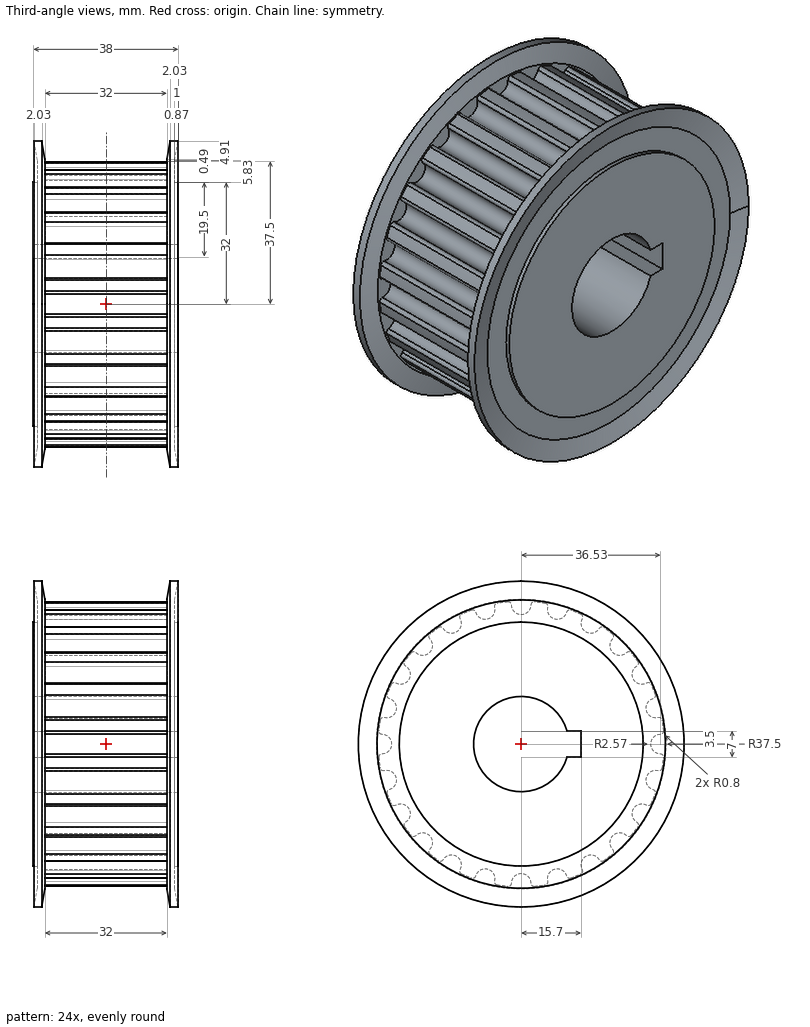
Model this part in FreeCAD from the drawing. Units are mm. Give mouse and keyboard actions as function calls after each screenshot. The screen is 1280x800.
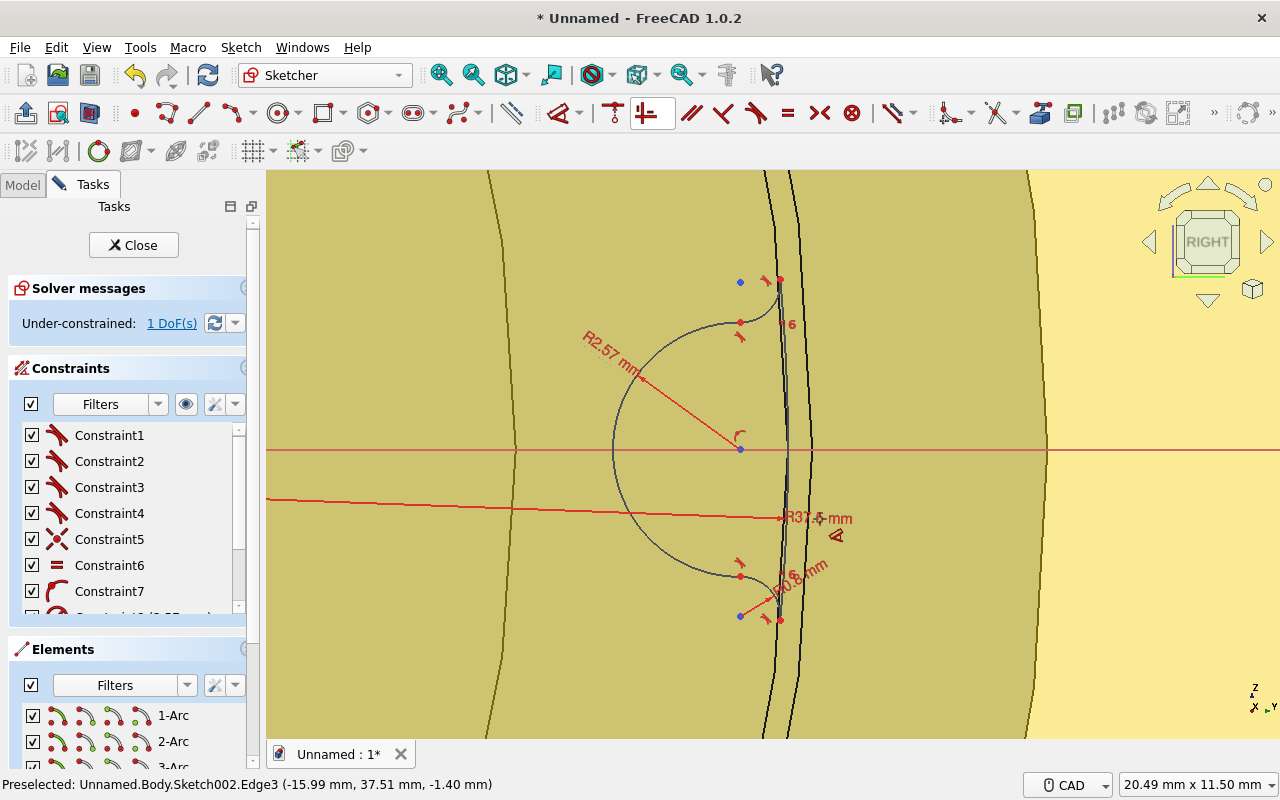
click(740, 450)
click(517, 484)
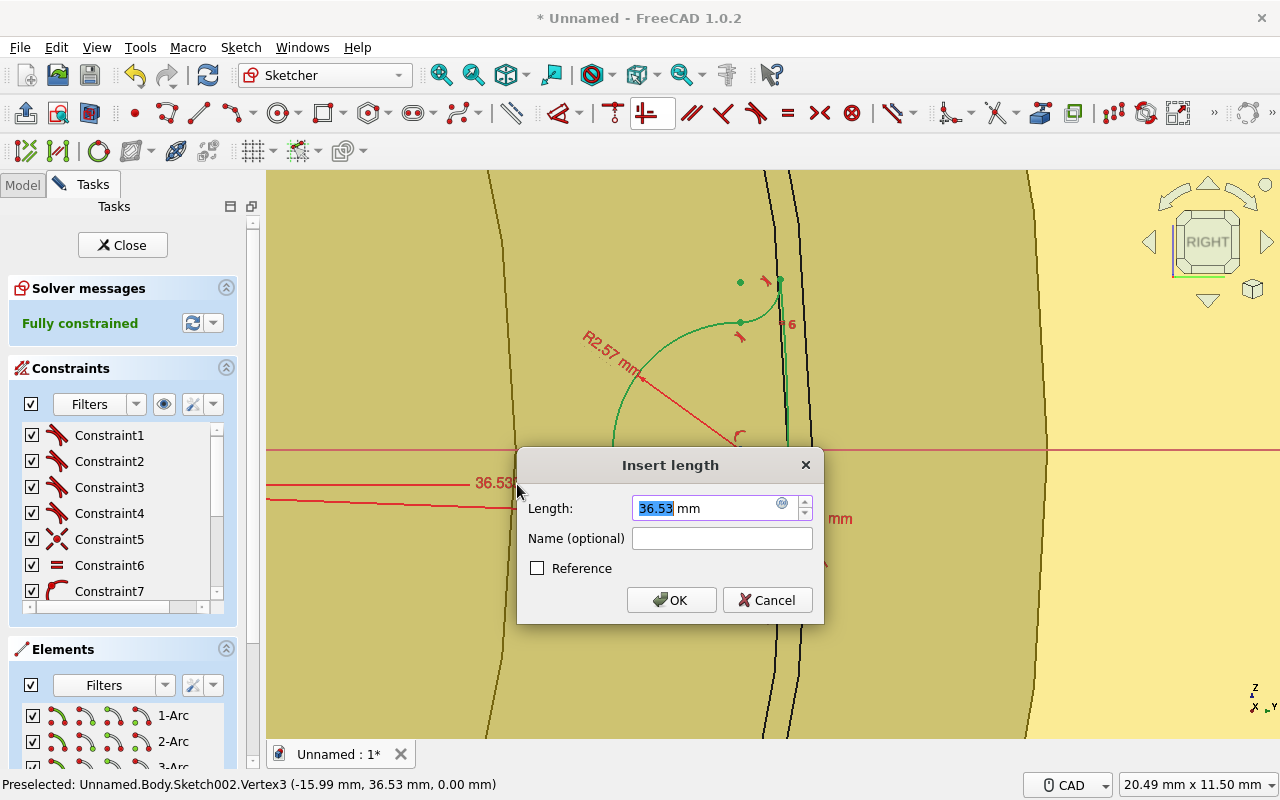
text(36.53)
key(Return)
key(Escape)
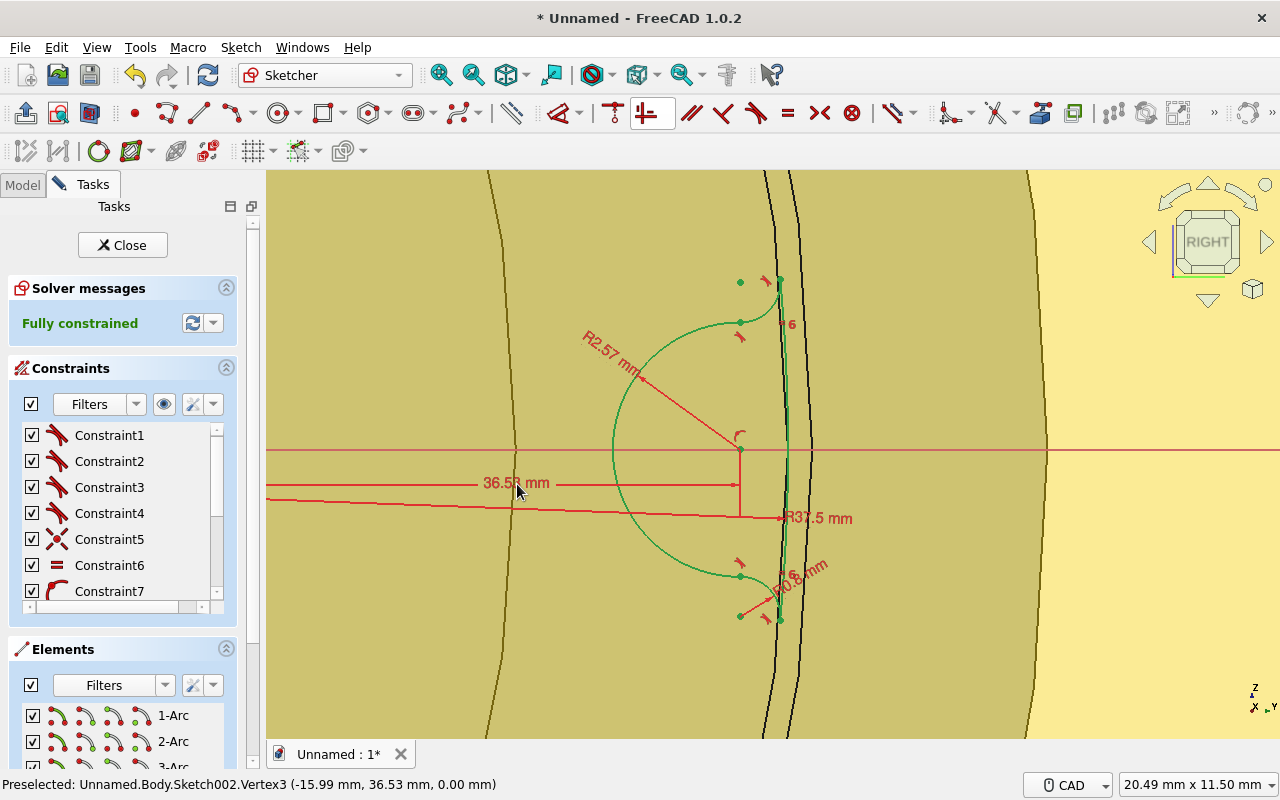
click(123, 245)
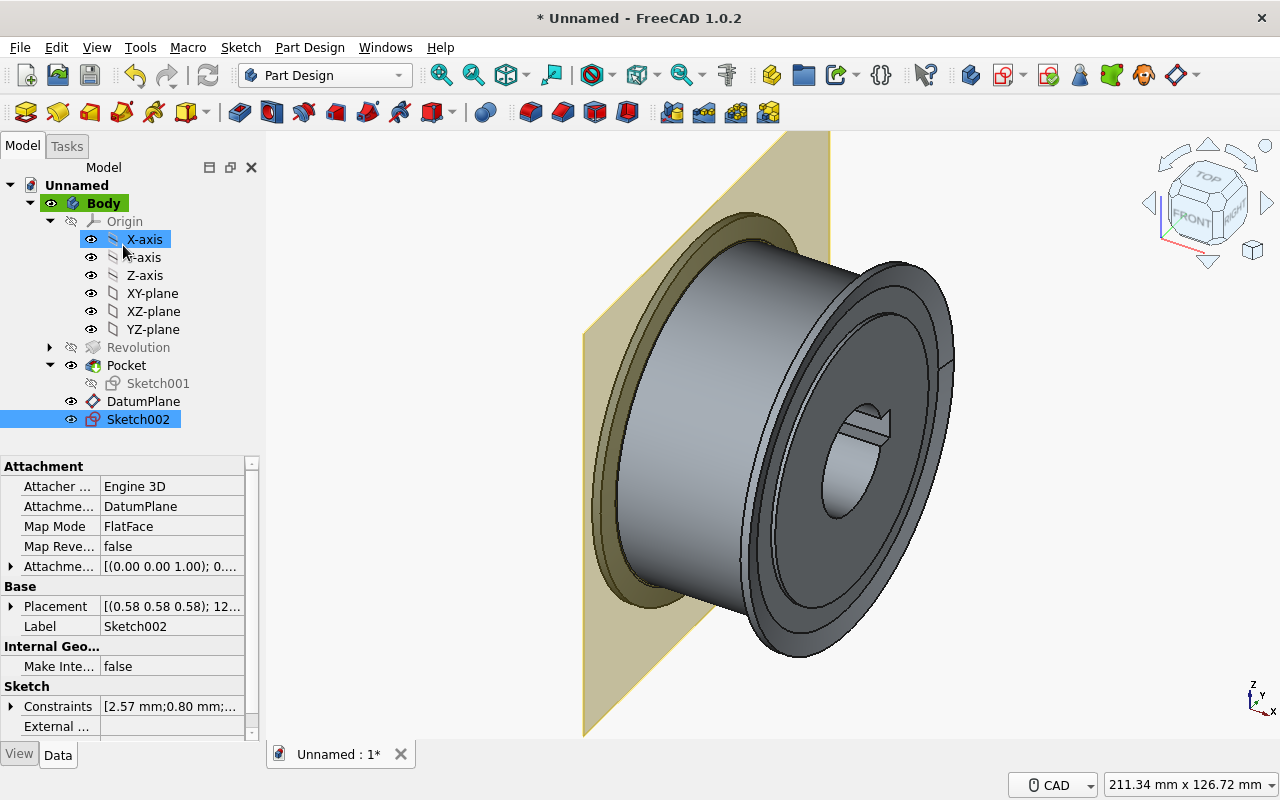
click(240, 112)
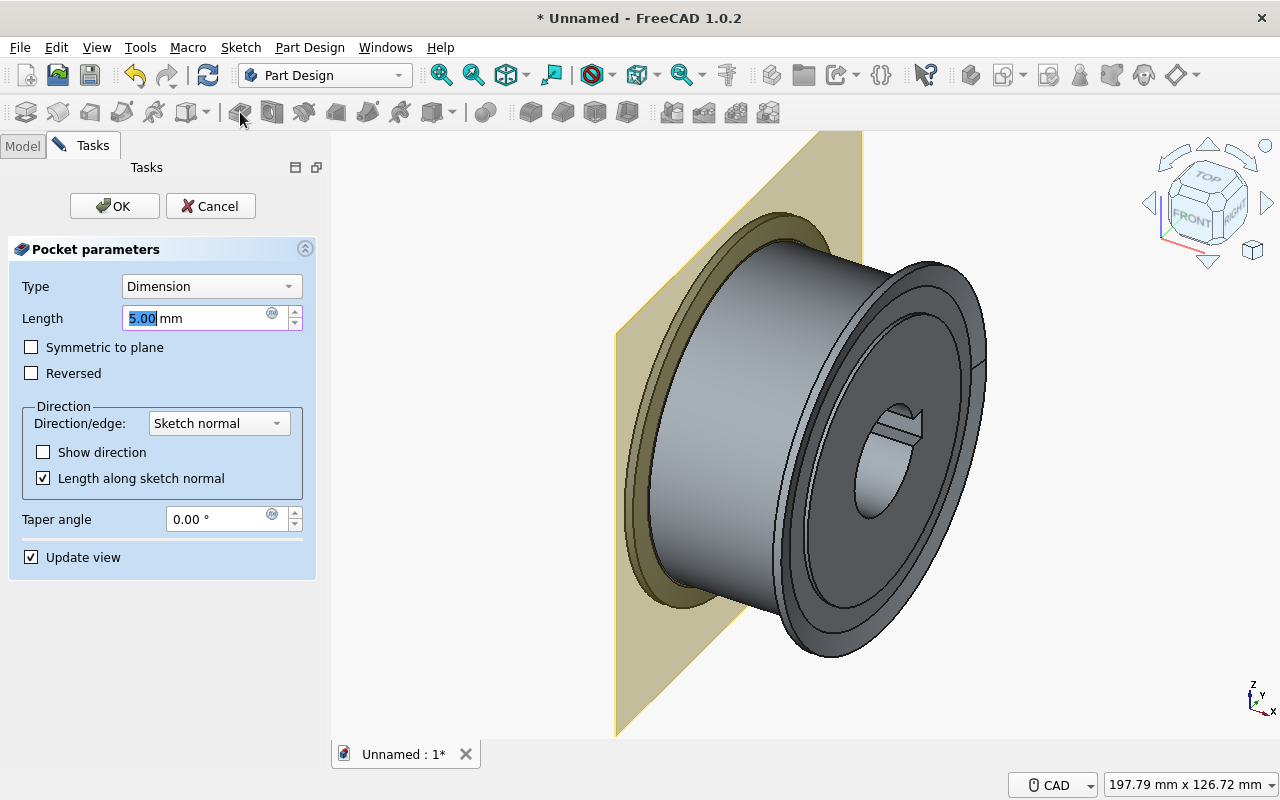
text(32)
key(Tab)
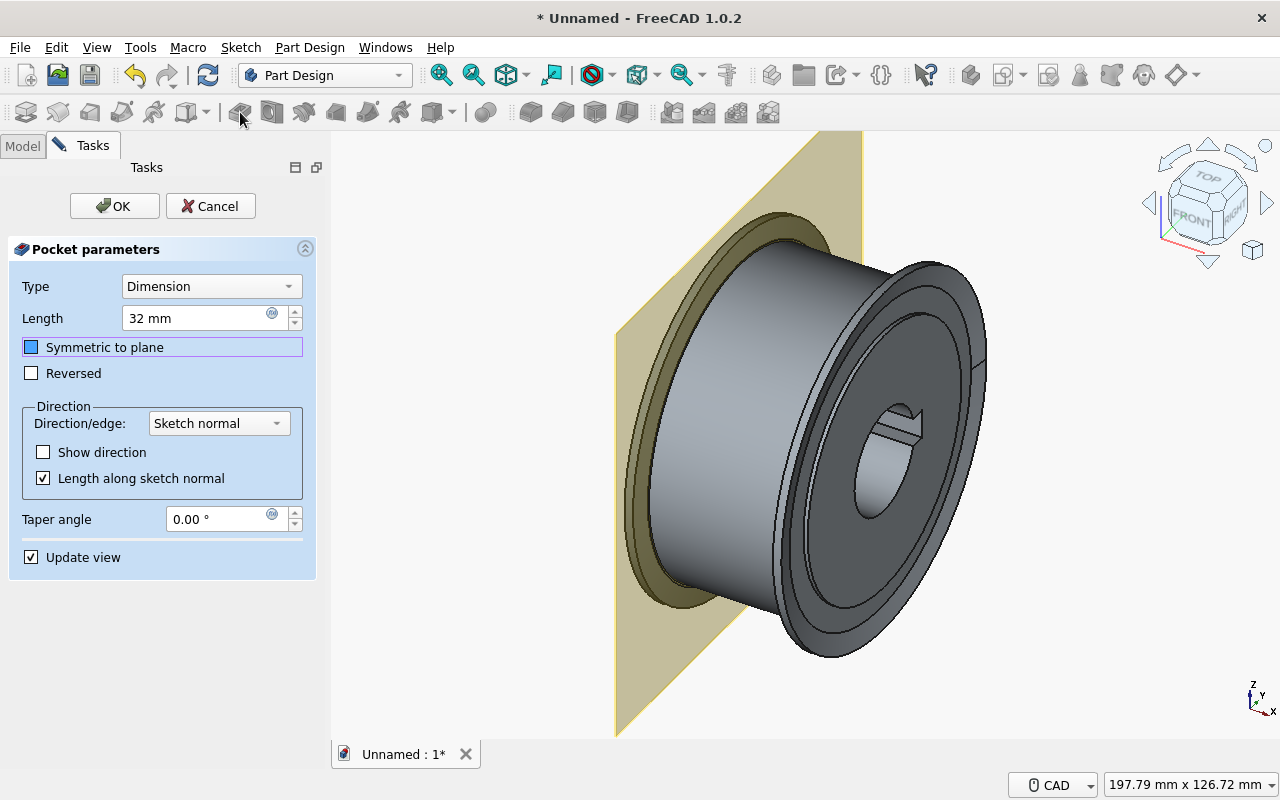
click(30, 373)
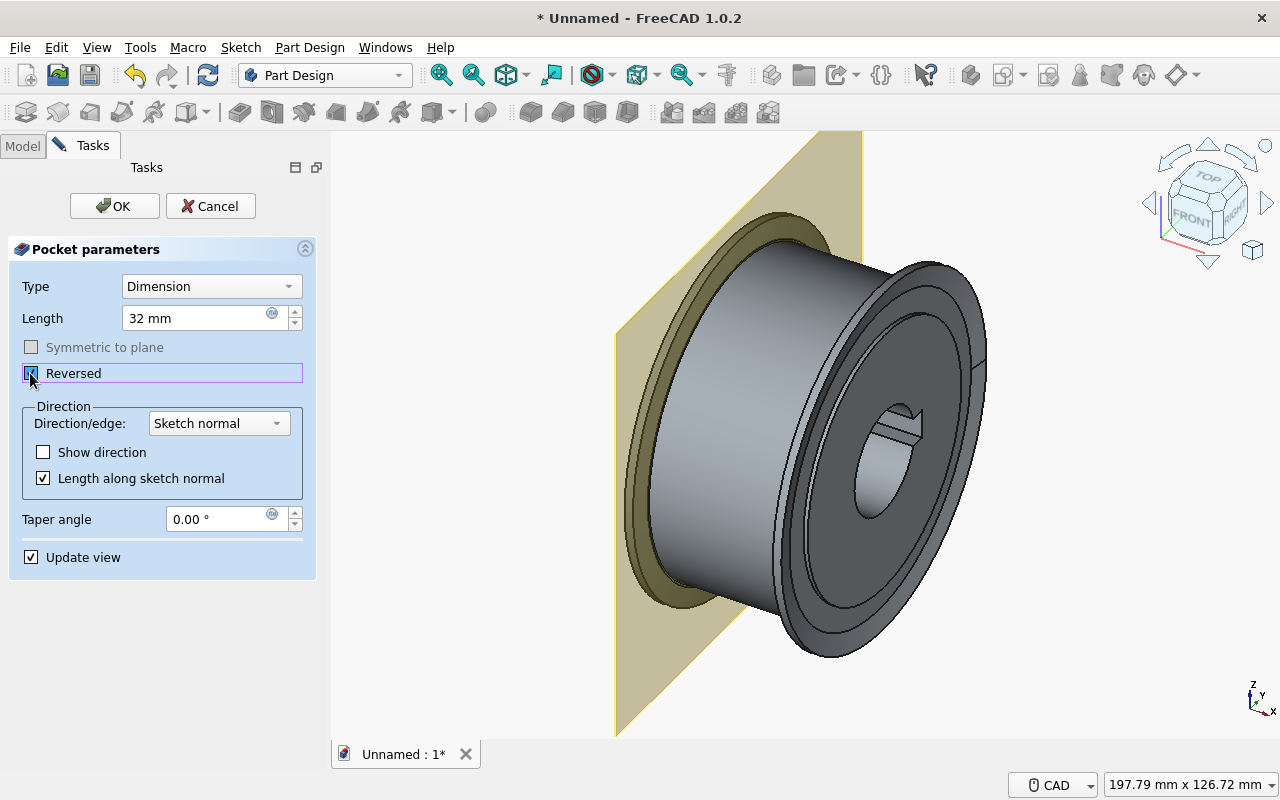
click(115, 206)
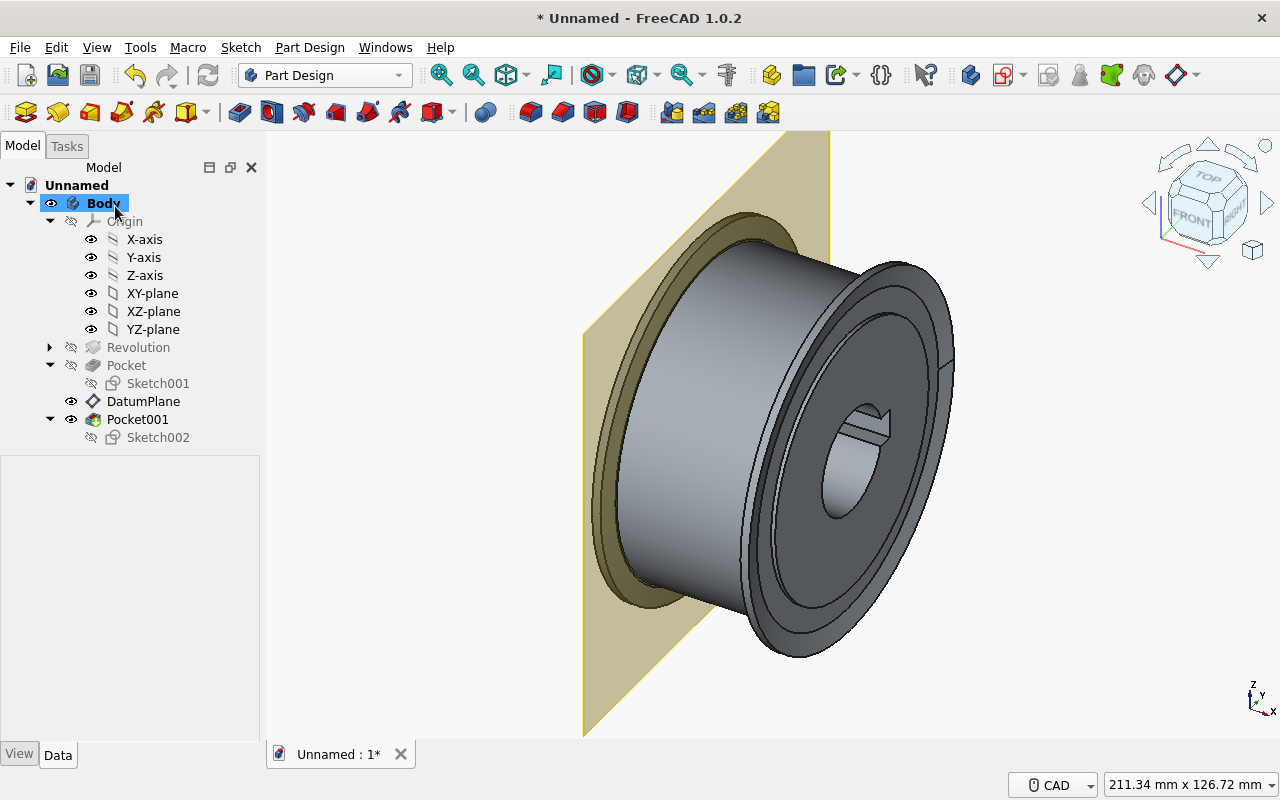
click(116, 401)
key(space)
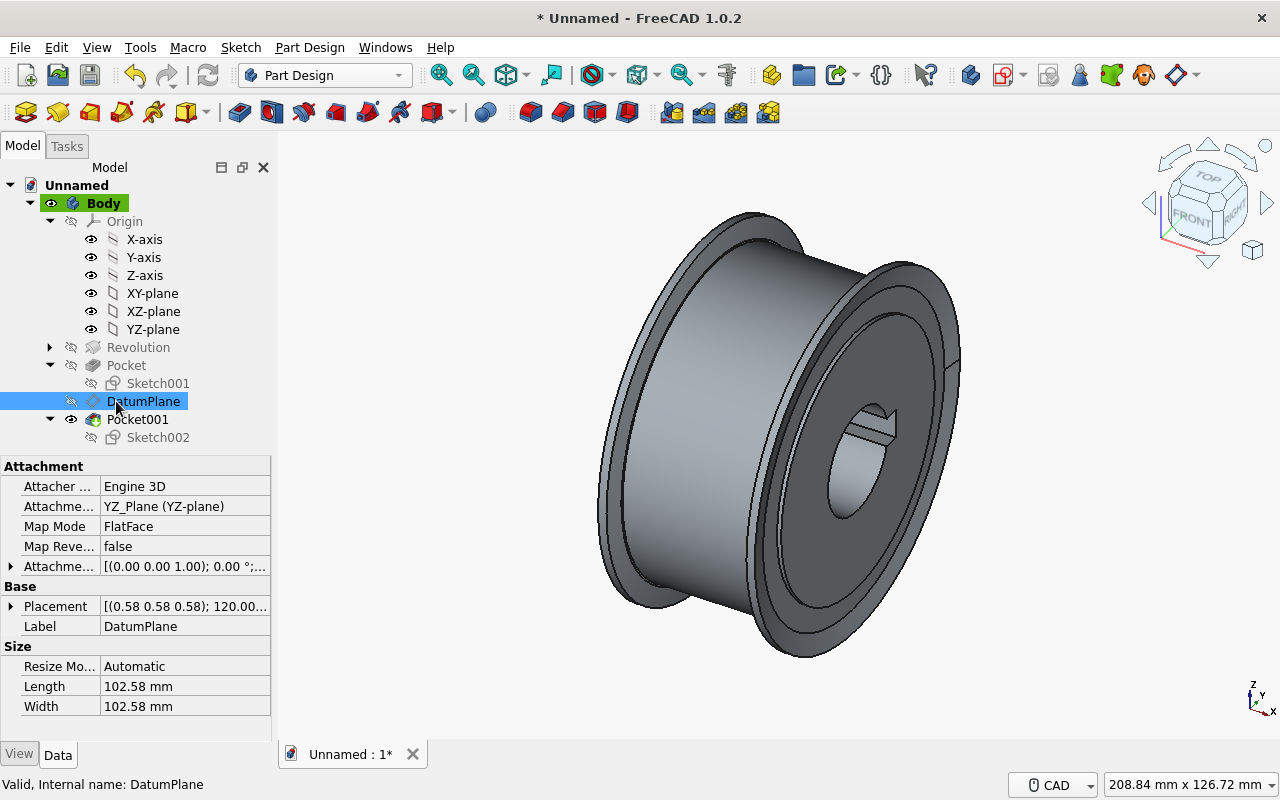
click(116, 419)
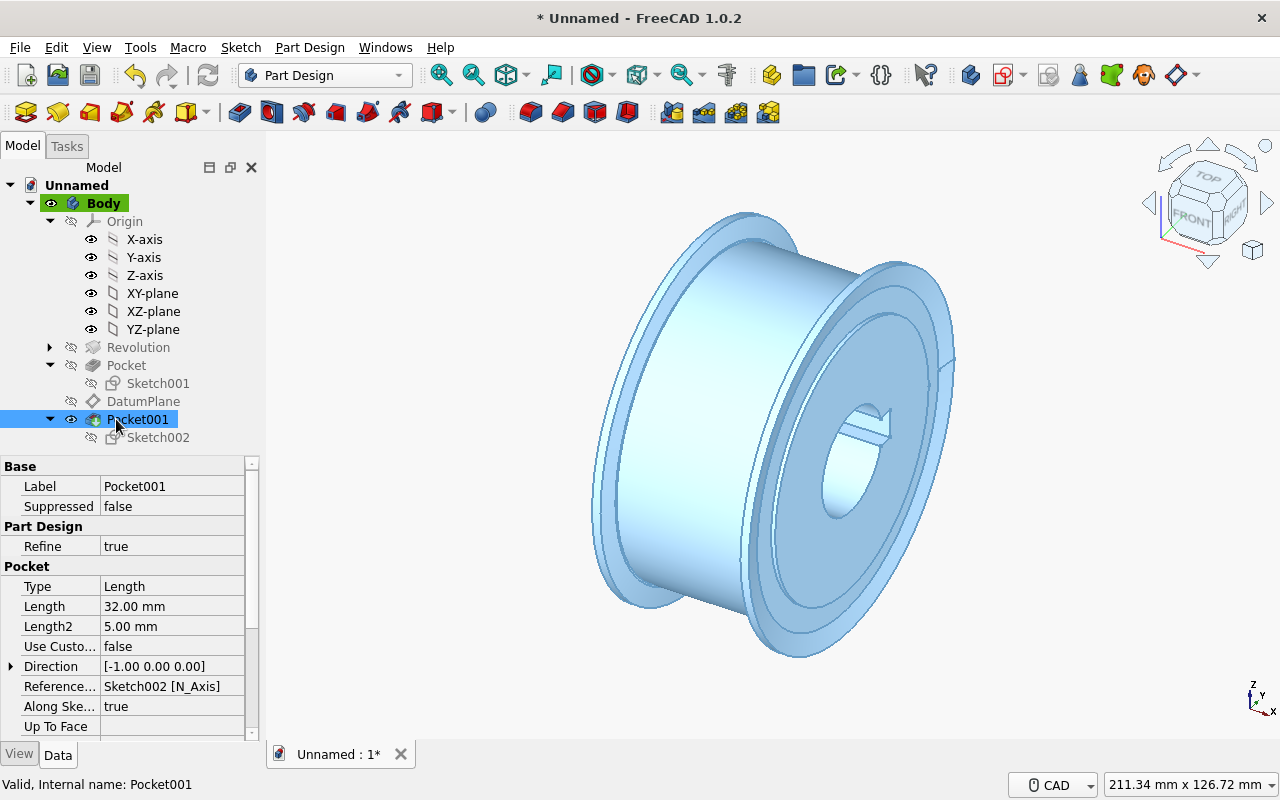
click(736, 112)